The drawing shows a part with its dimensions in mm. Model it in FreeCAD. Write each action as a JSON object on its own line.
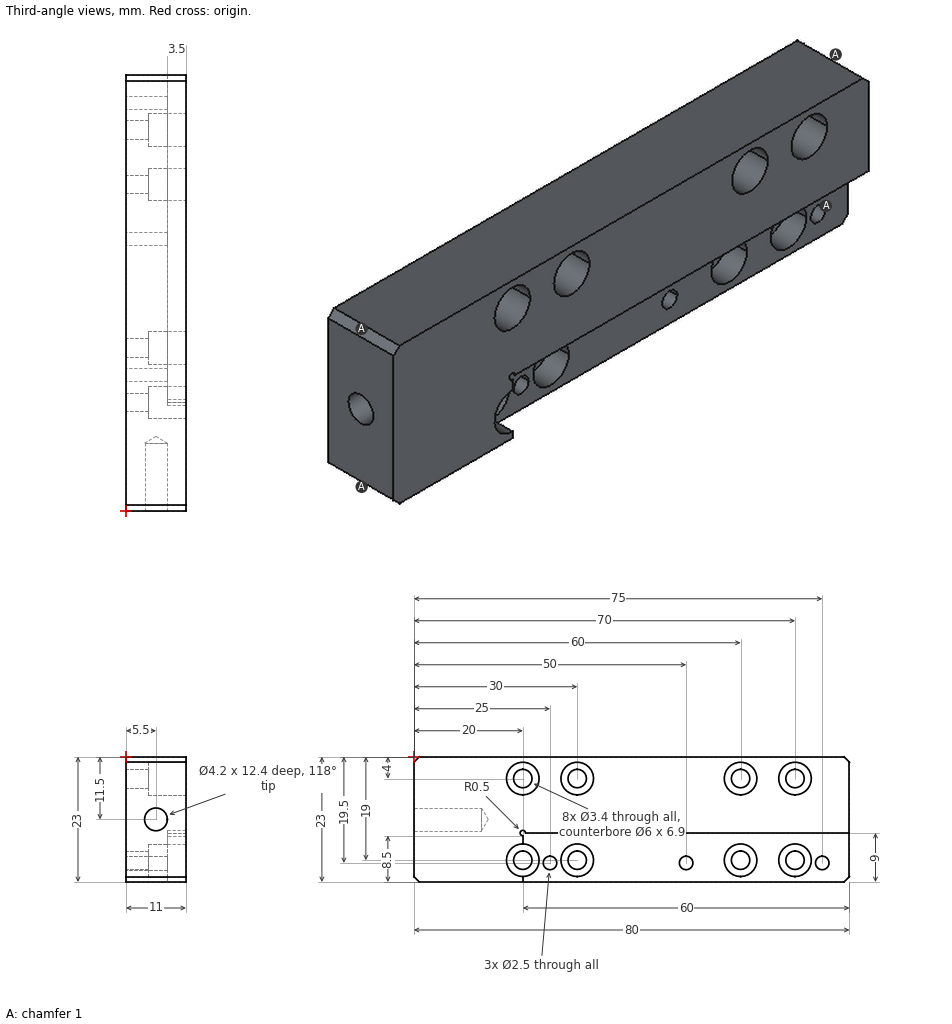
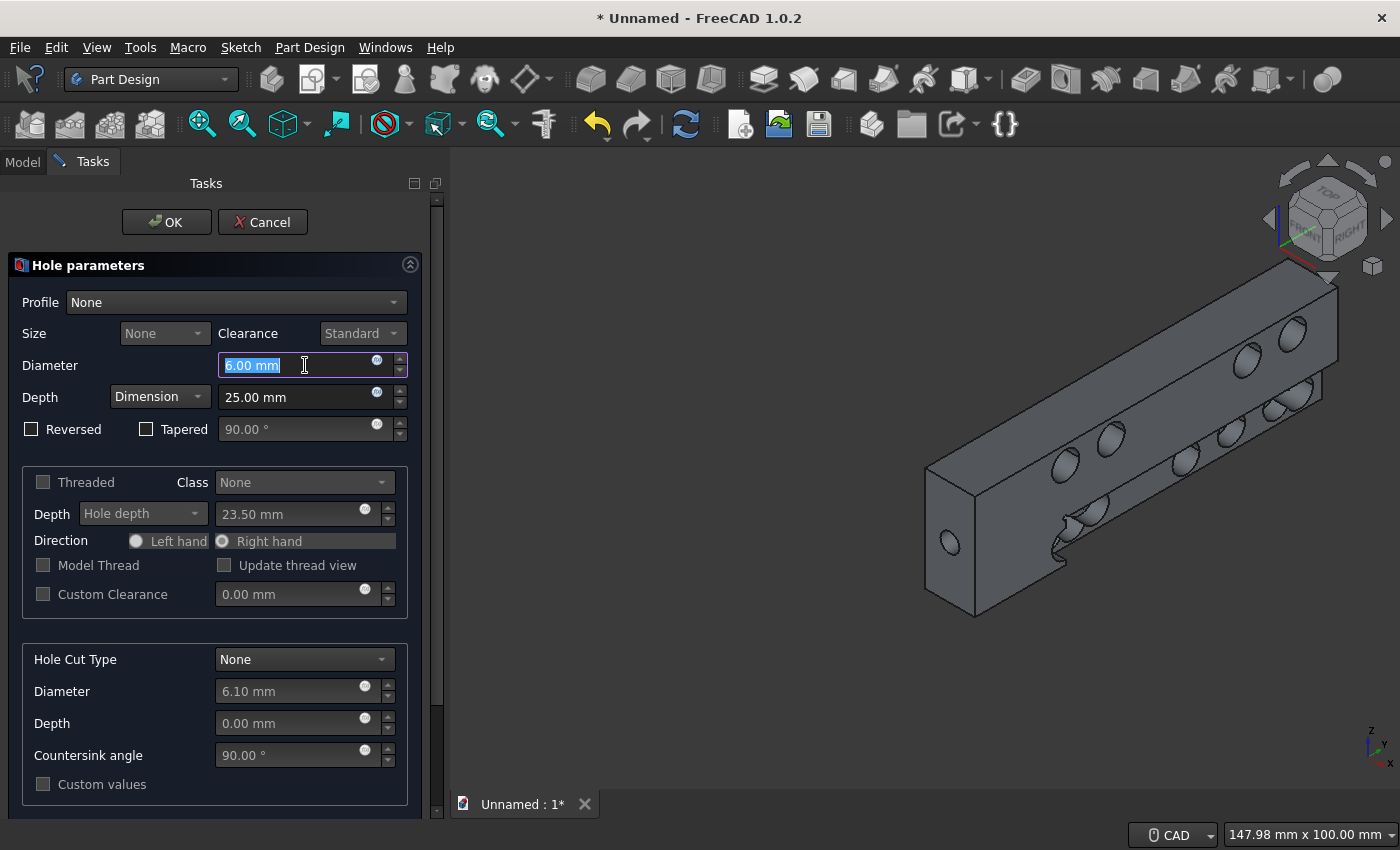
{"action": "type", "text": "2.5"}
{"action": "key", "text": "Tab"}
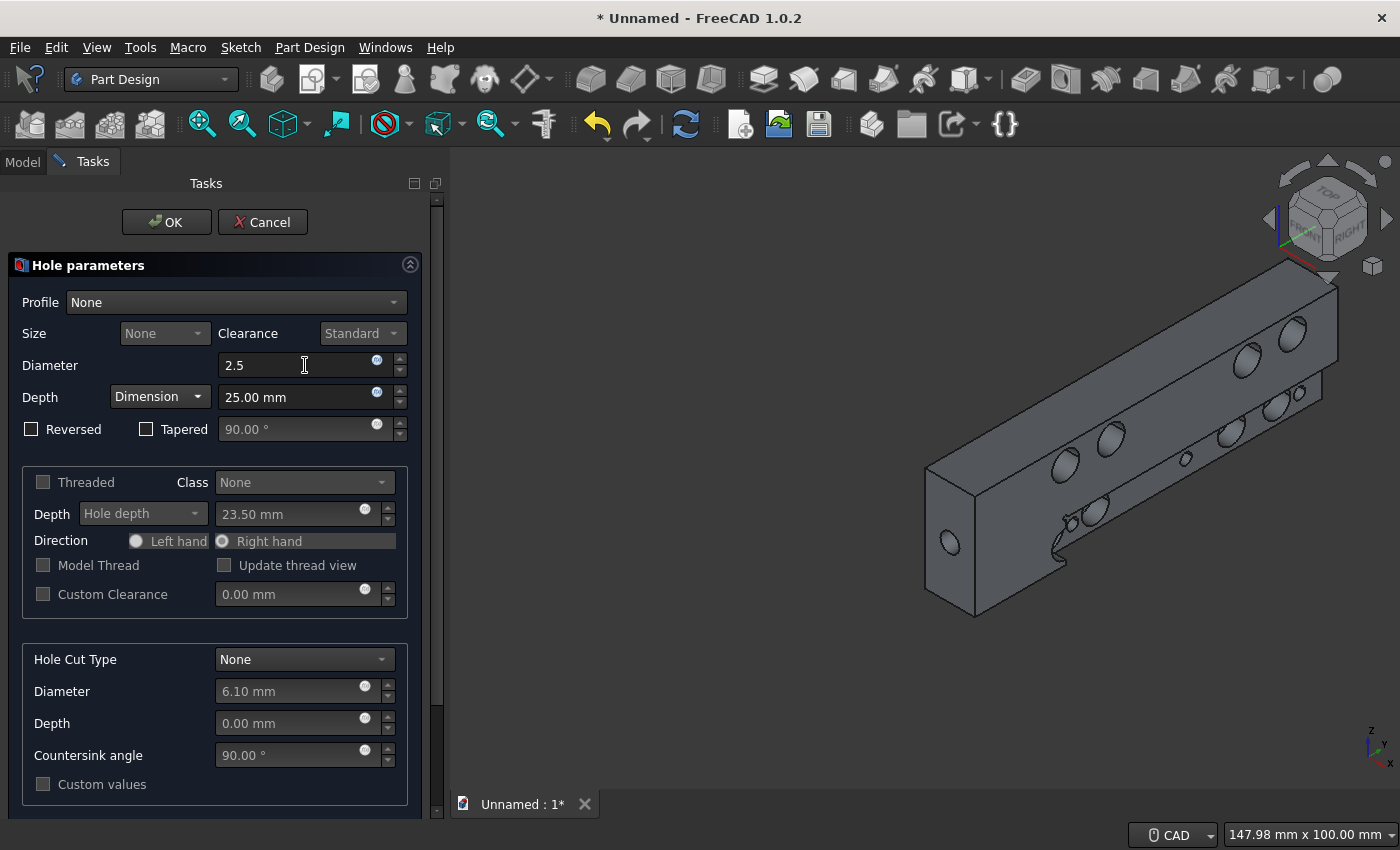
{"action": "left_click", "coordinate": [161, 396]}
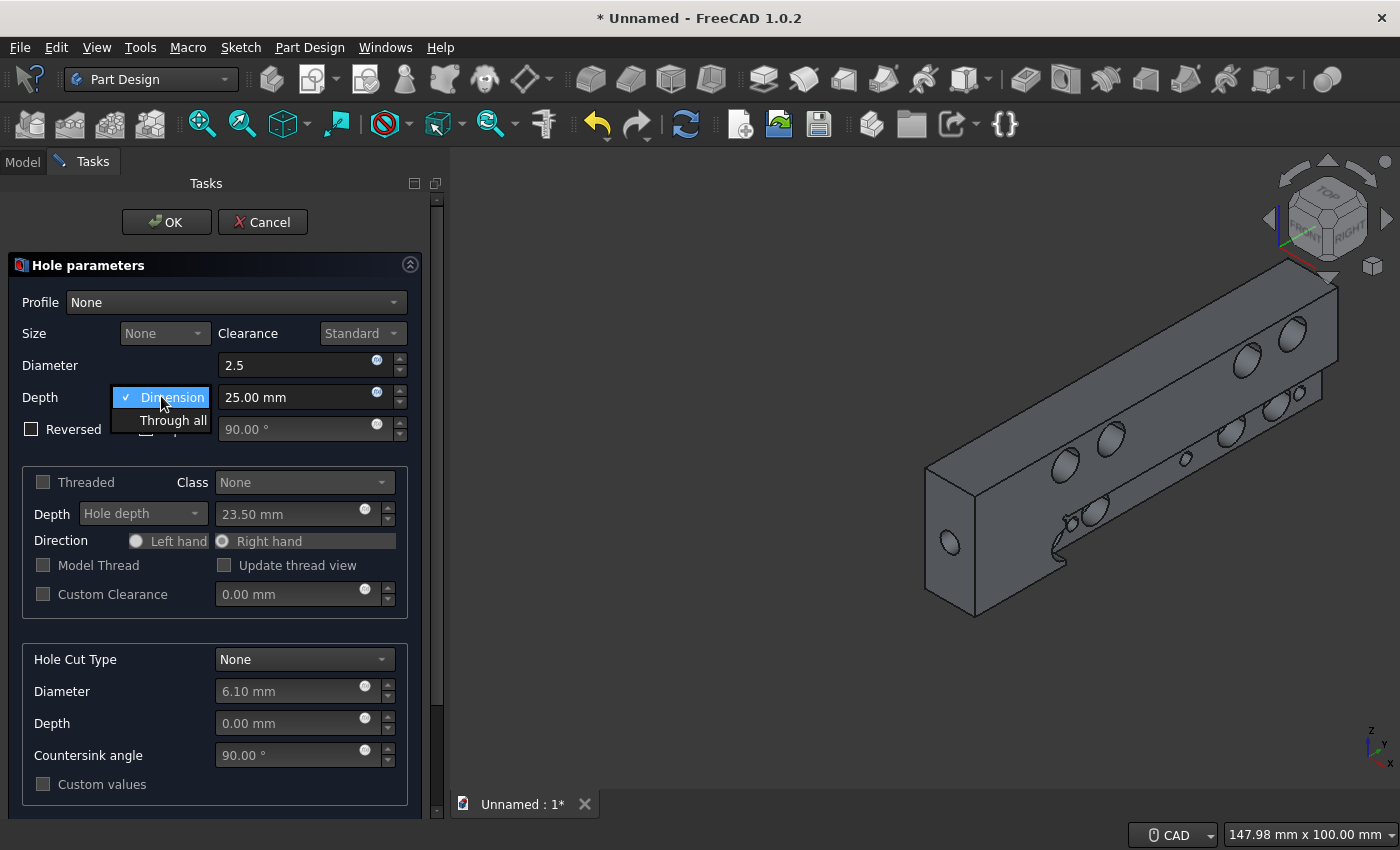
{"action": "left_click", "coordinate": [160, 420]}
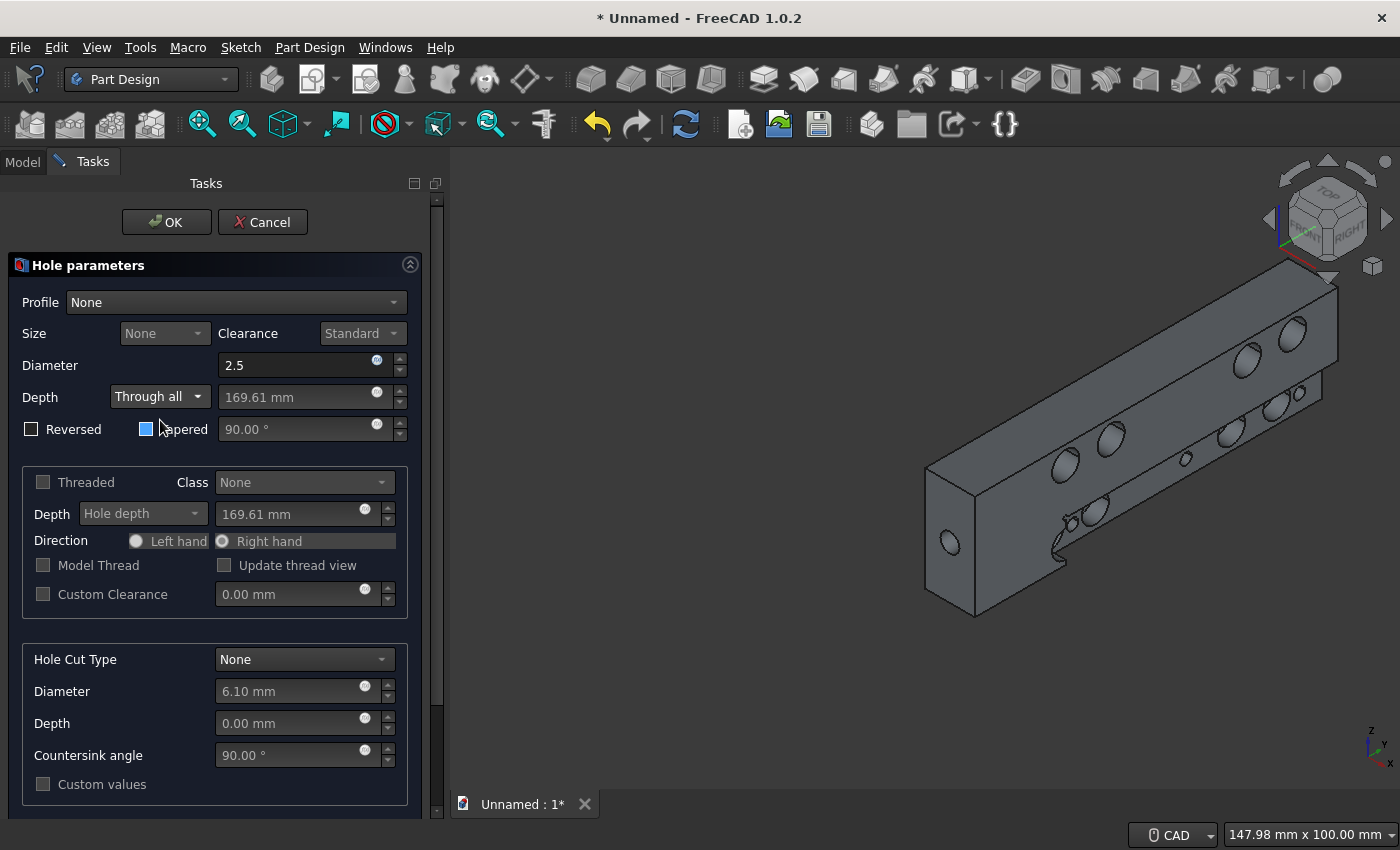
{"action": "left_click", "coordinate": [167, 222]}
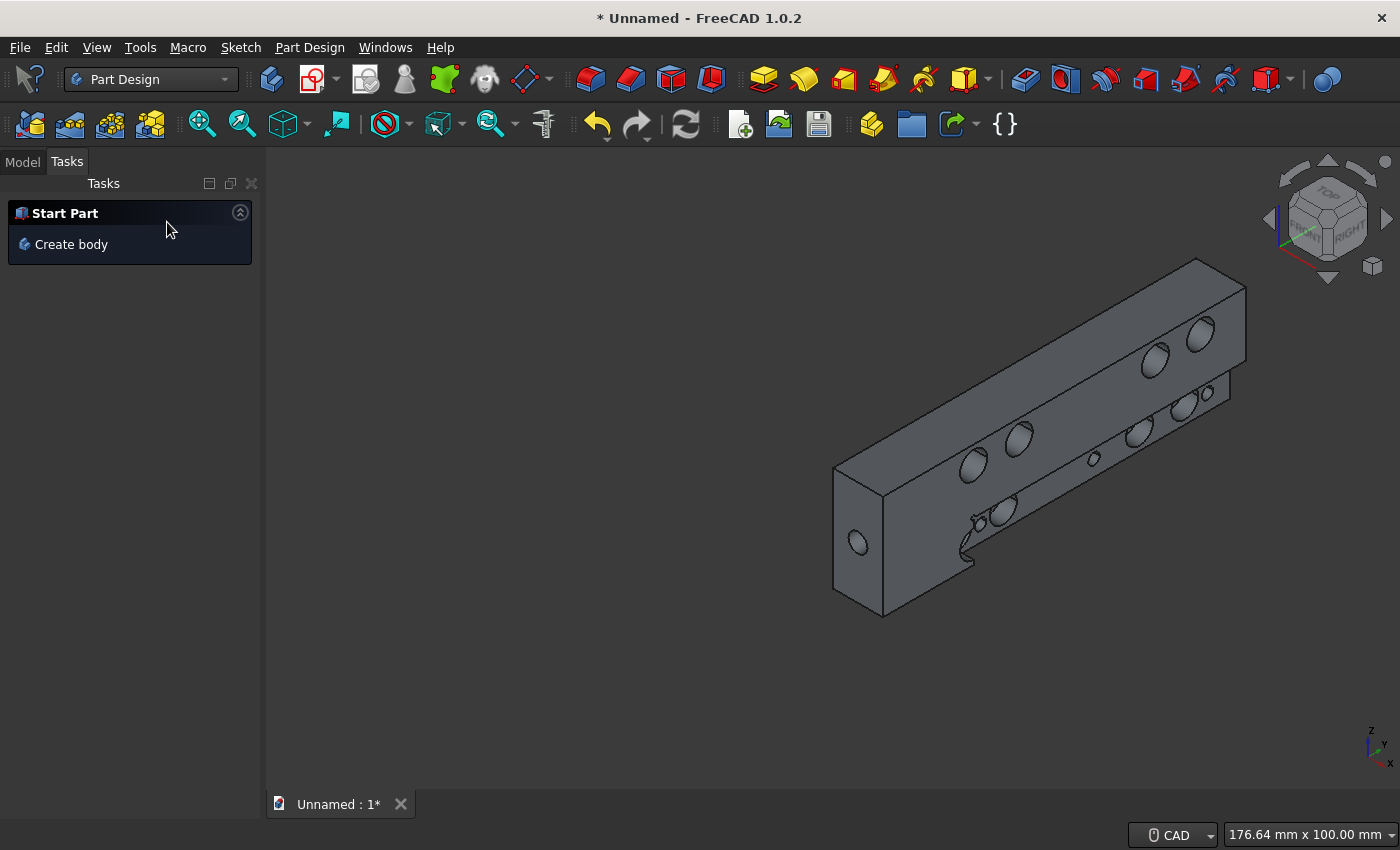
{"action": "left_click", "coordinate": [858, 481]}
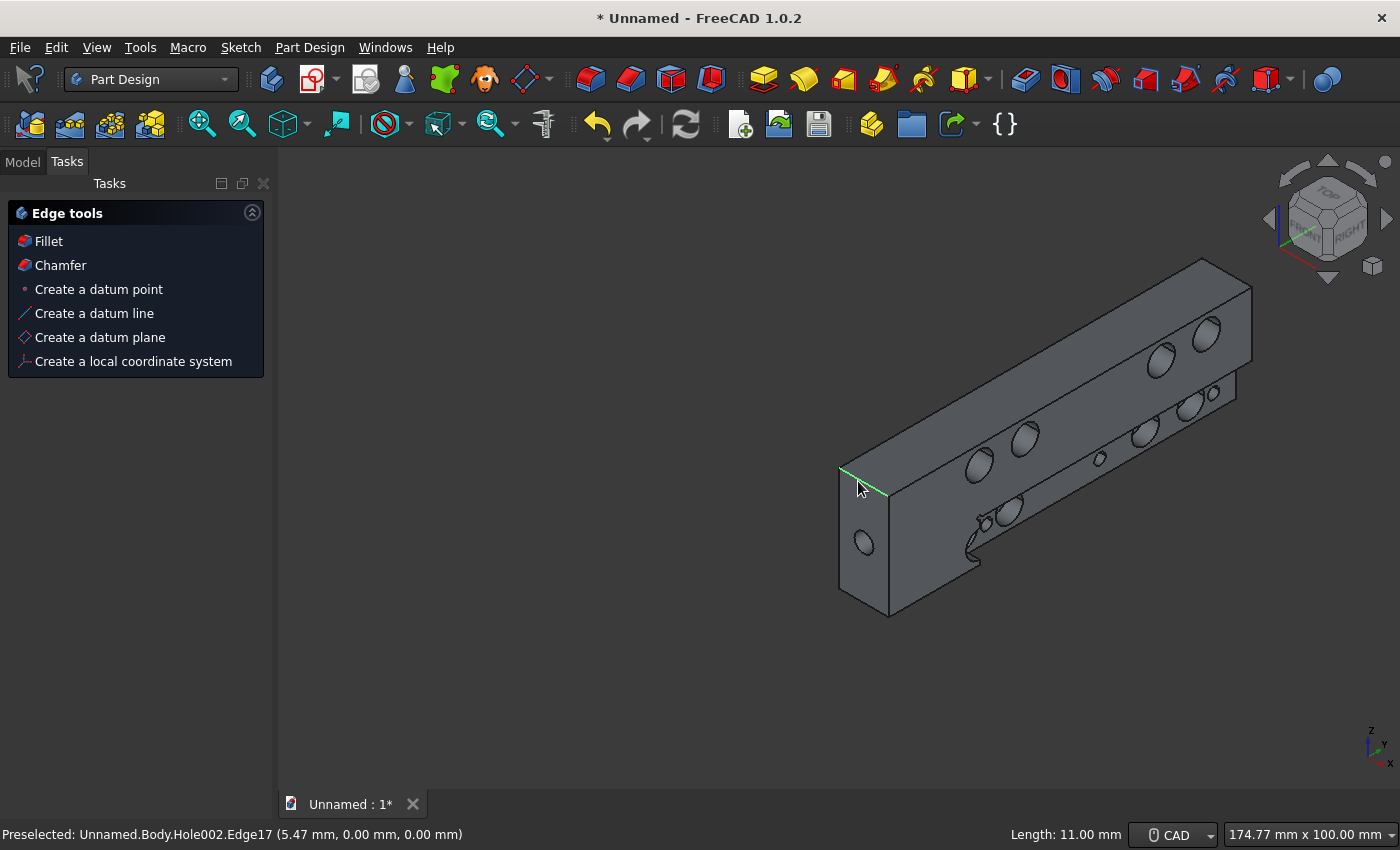
{"action": "key", "text": "2"}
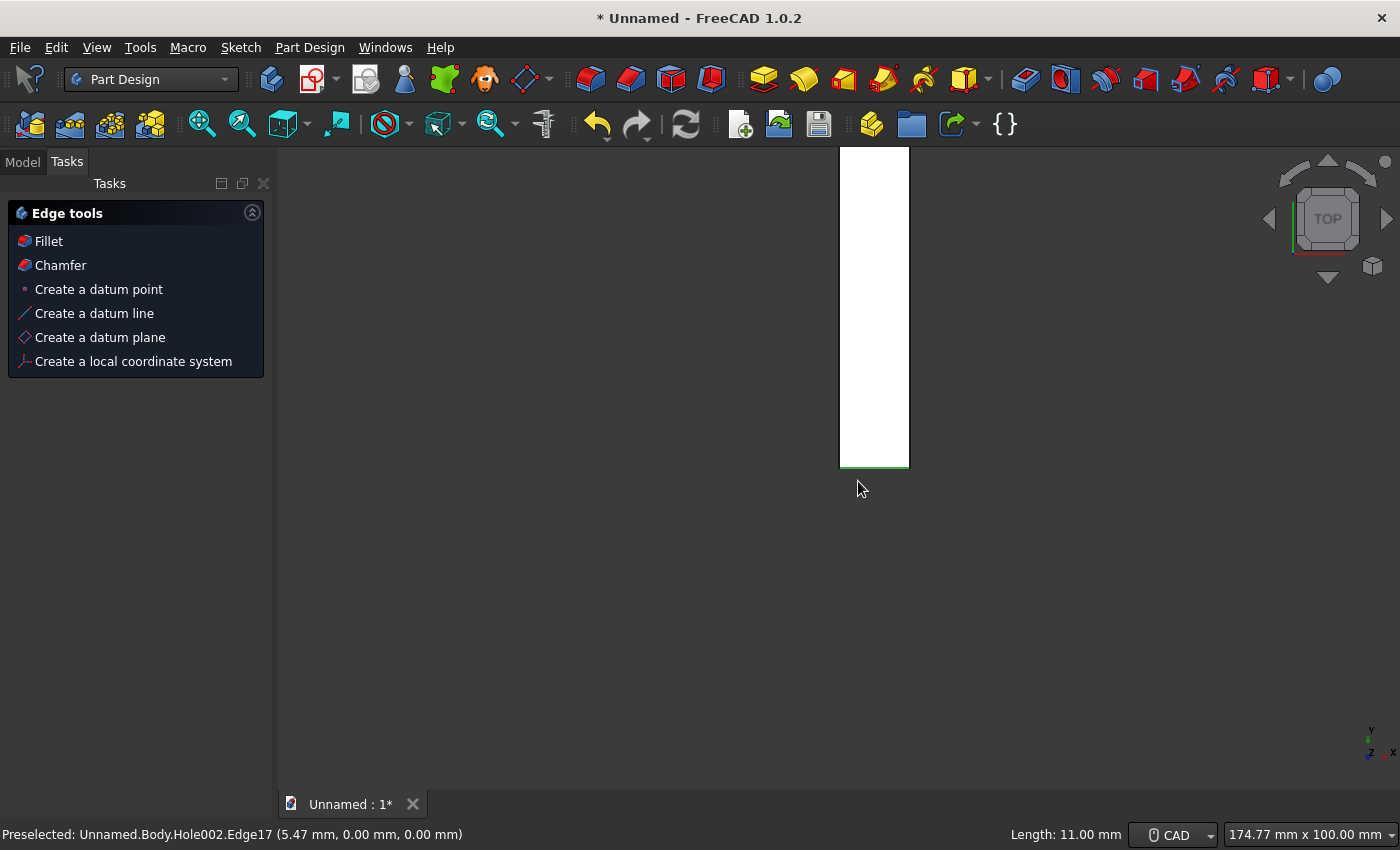
{"action": "left_click", "coordinate": [204, 124]}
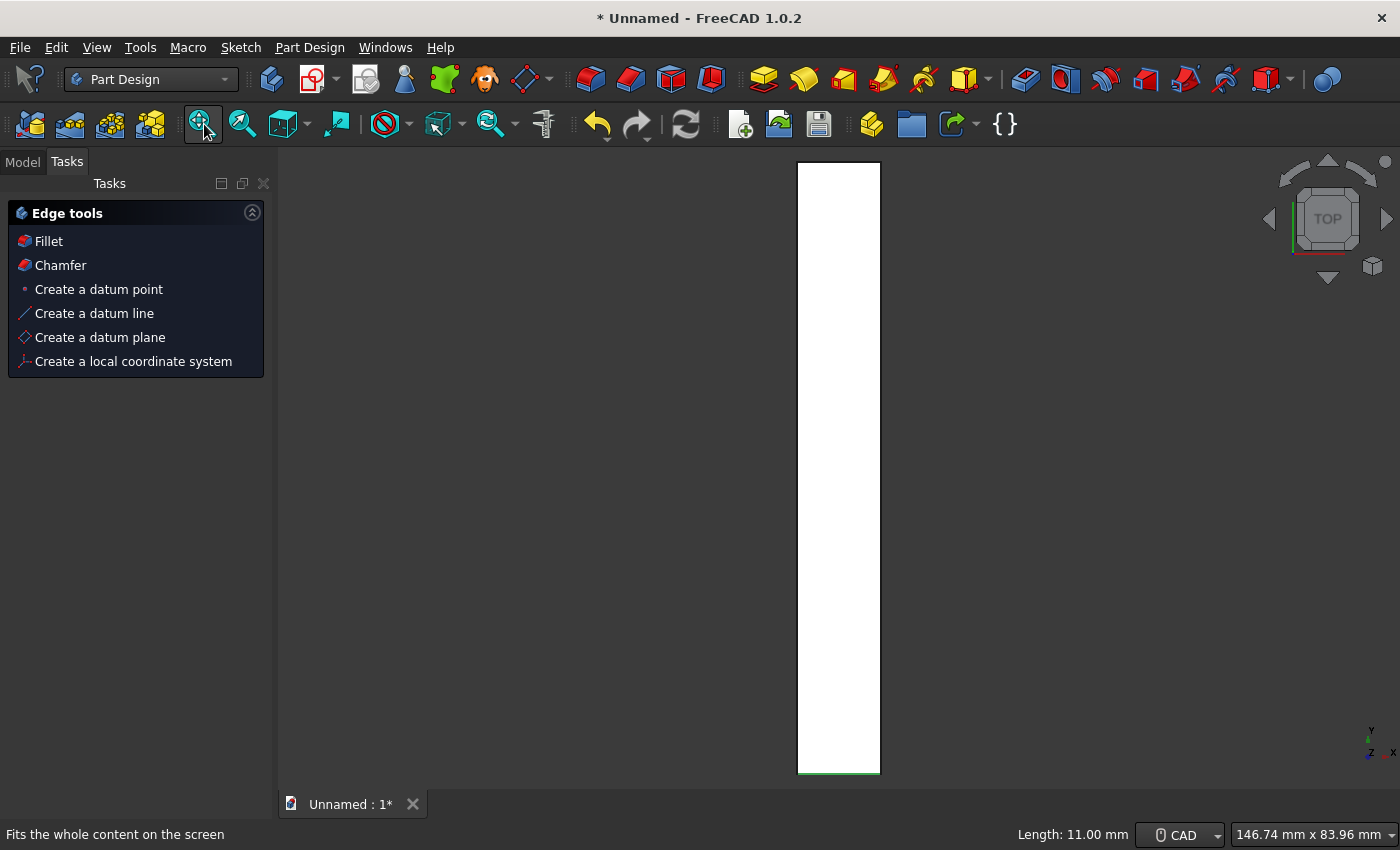
{"action": "key", "text": "0"}